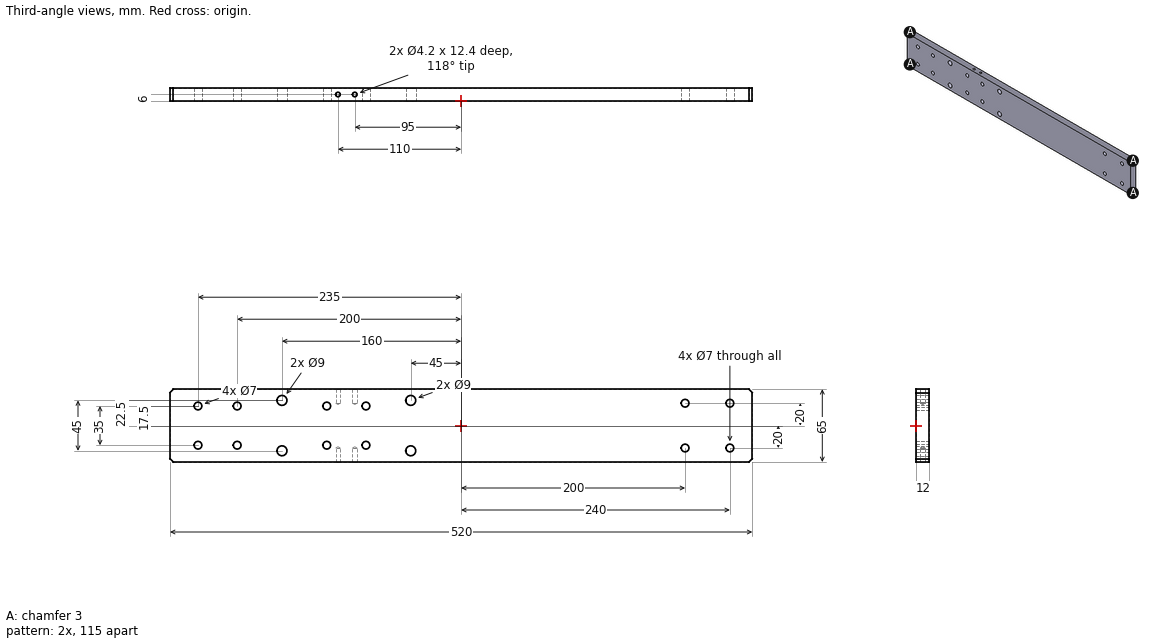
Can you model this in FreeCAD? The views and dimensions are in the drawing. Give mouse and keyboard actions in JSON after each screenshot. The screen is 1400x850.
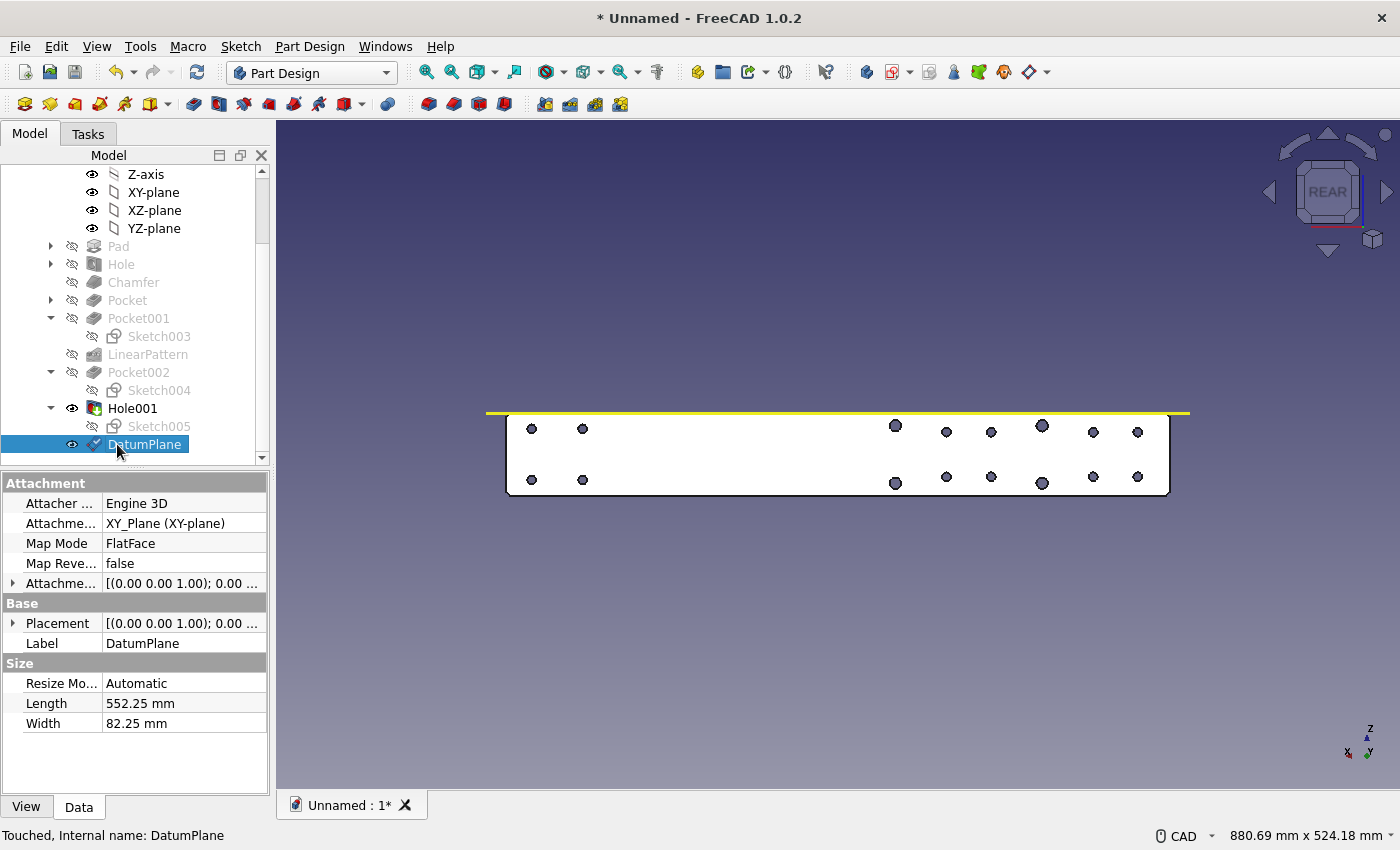
{"action": "left_click", "coordinate": [892, 72]}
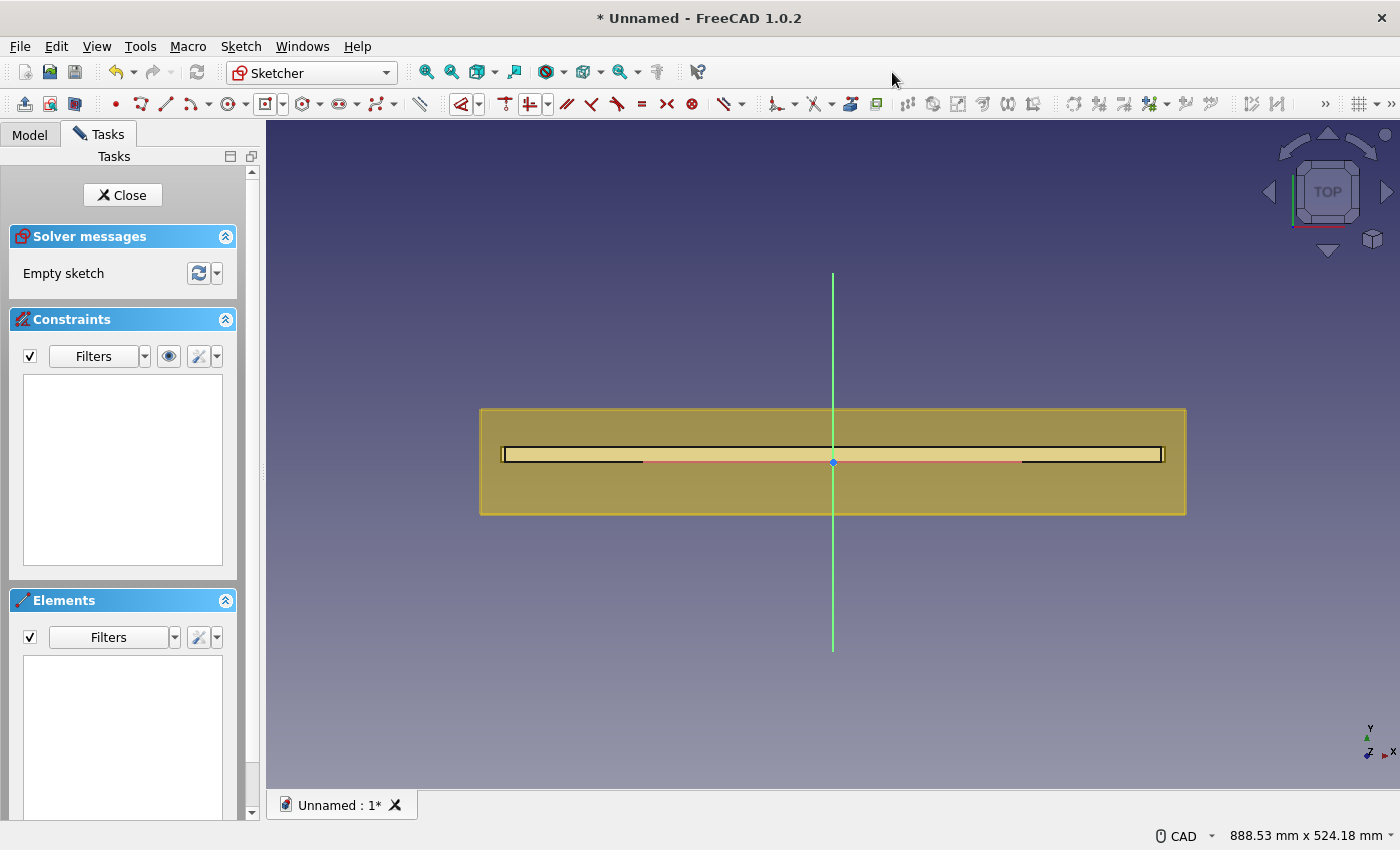
{"action": "scroll", "coordinate": [699, 454], "scroll_direction": "up", "scroll_amount": 15}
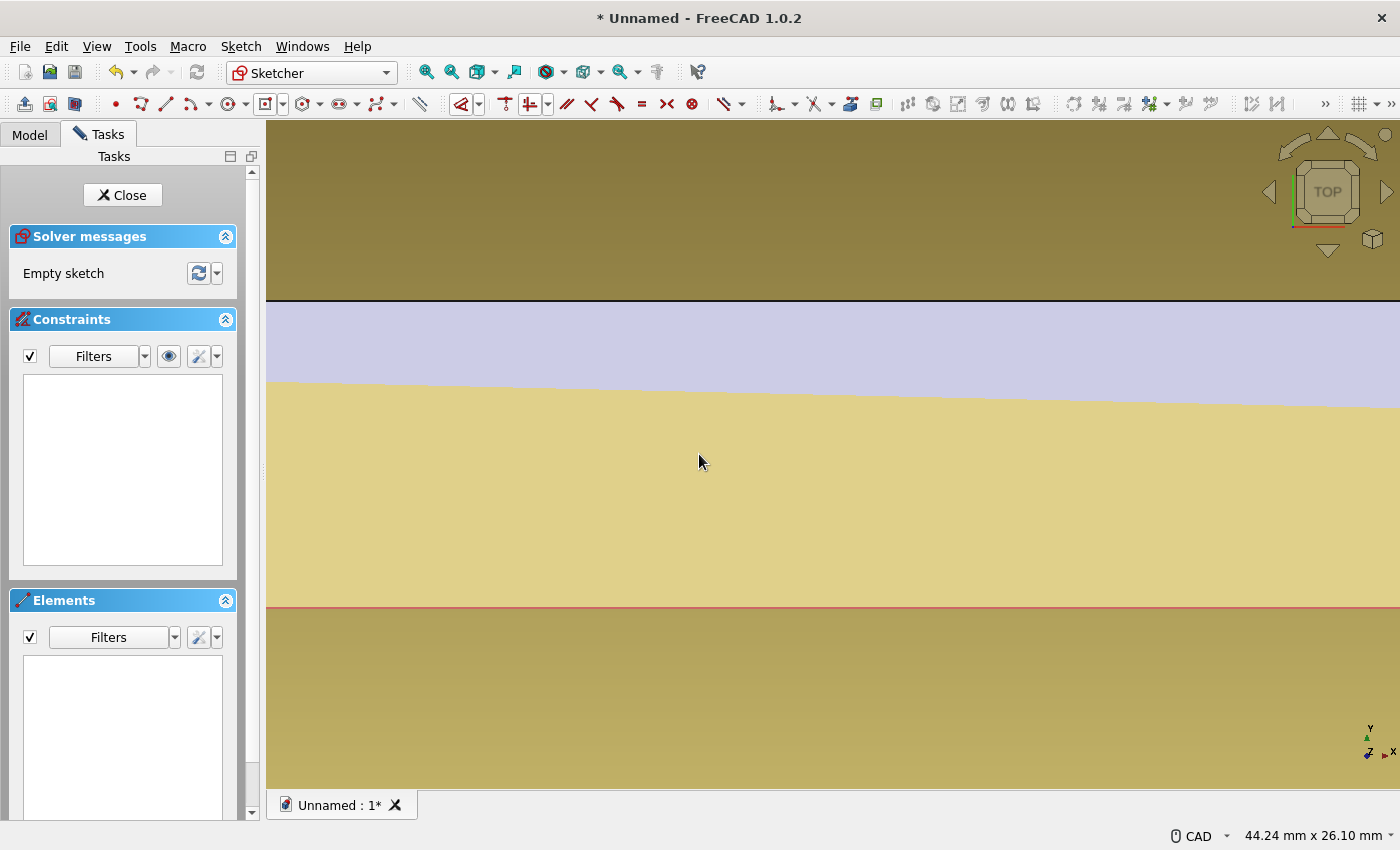
{"action": "left_click", "coordinate": [228, 104]}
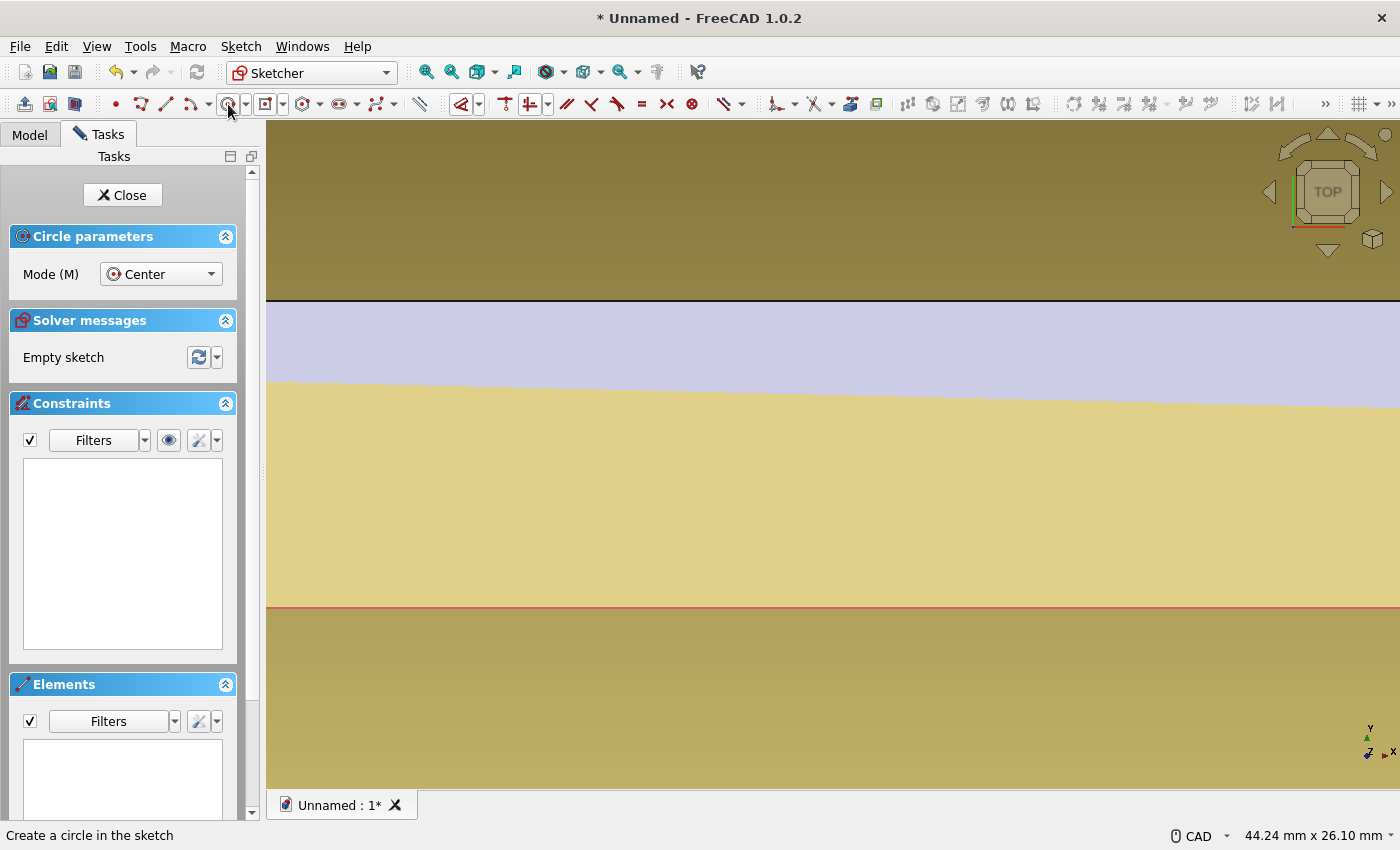
{"action": "left_click", "coordinate": [948, 454]}
{"action": "left_click", "coordinate": [986, 416]}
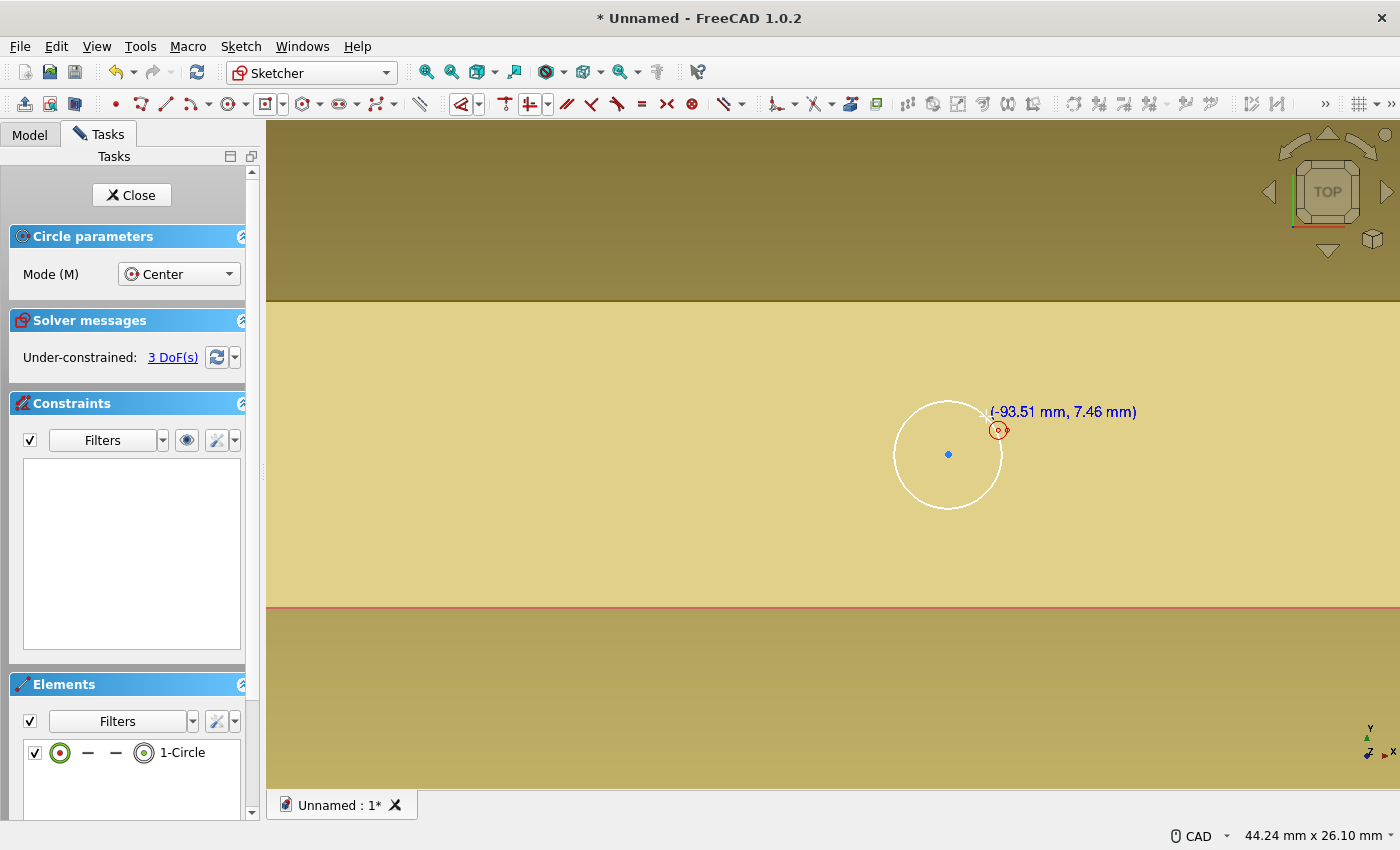
{"action": "left_click", "coordinate": [563, 454]}
{"action": "left_click", "coordinate": [601, 416]}
{"action": "key", "text": "Escape"}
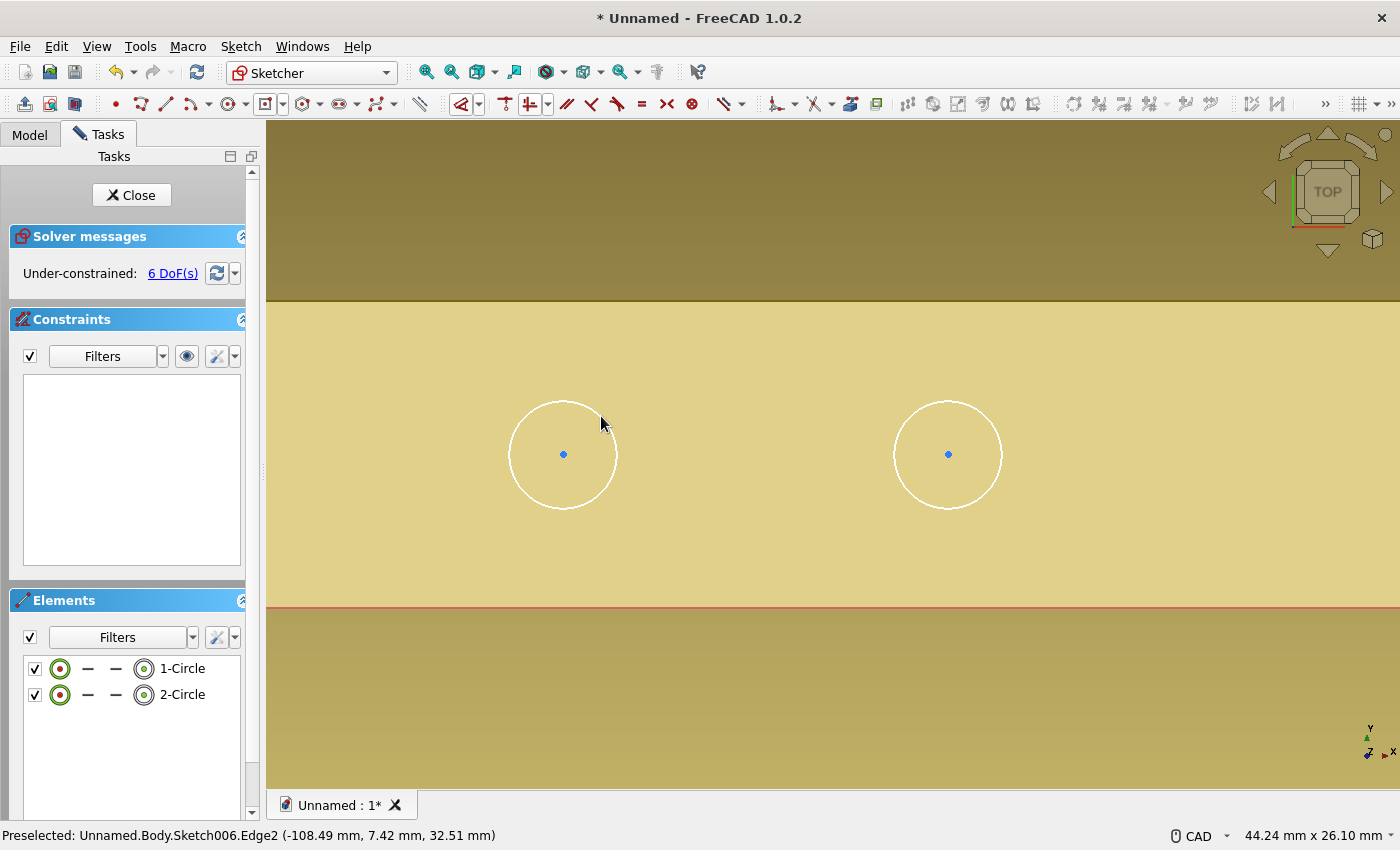
{"action": "left_click", "coordinate": [986, 417]}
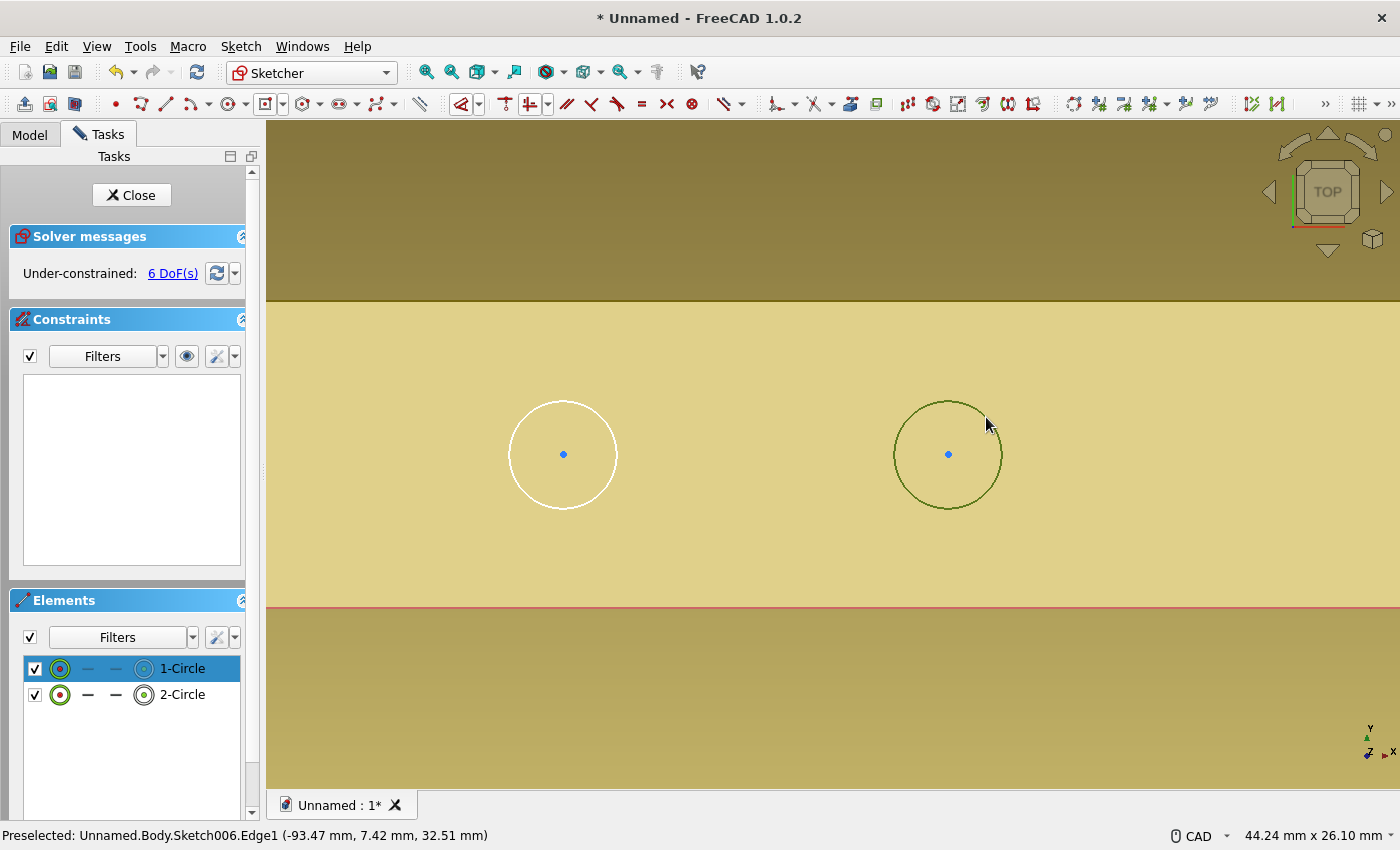
{"action": "left_click", "coordinate": [601, 417]}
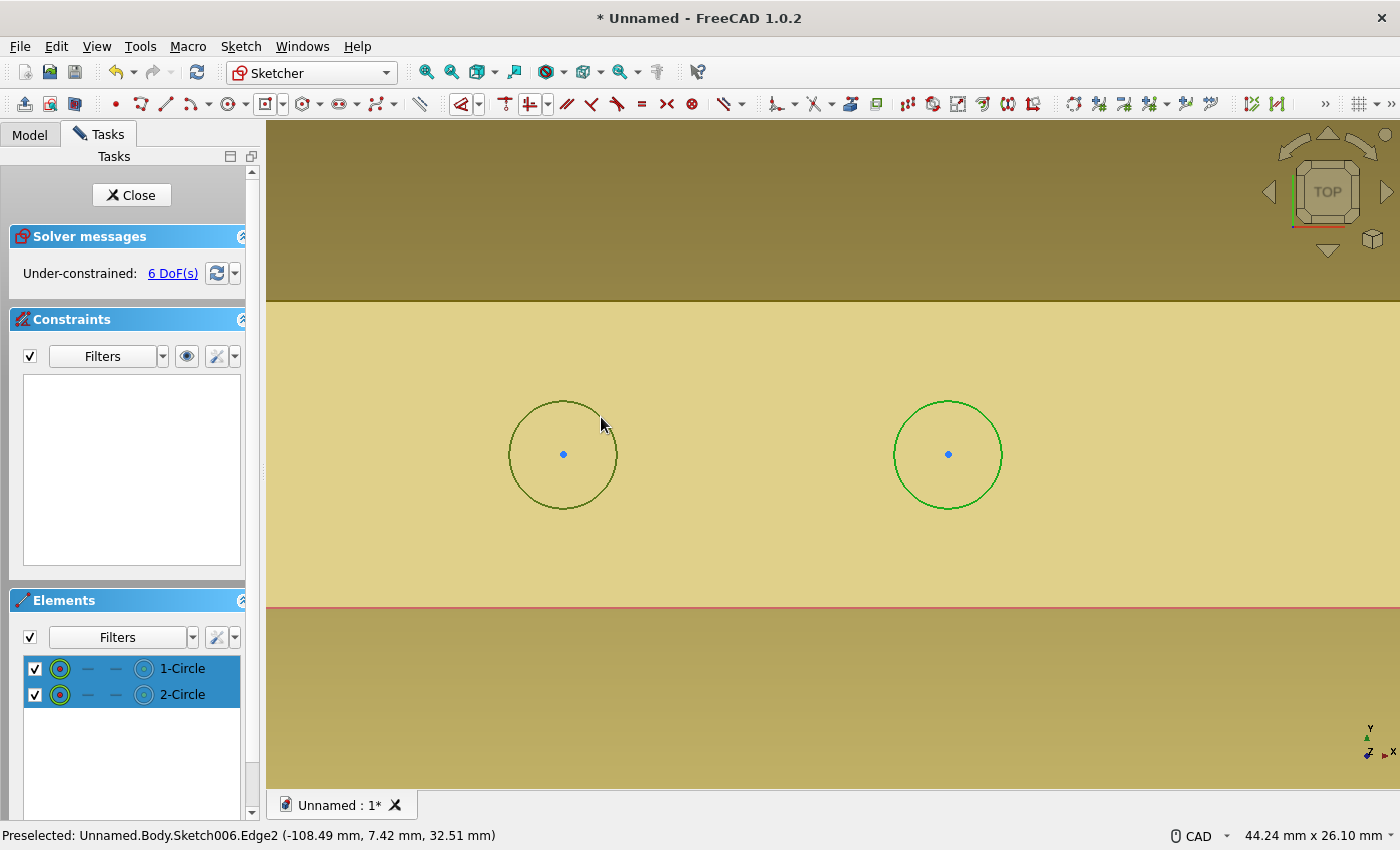
{"action": "left_click", "coordinate": [642, 104]}